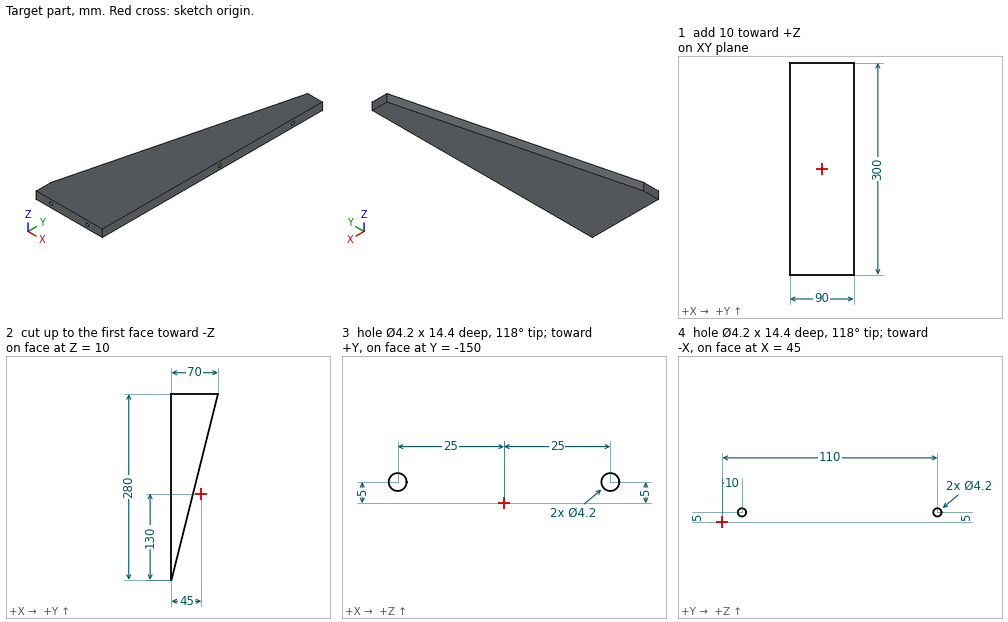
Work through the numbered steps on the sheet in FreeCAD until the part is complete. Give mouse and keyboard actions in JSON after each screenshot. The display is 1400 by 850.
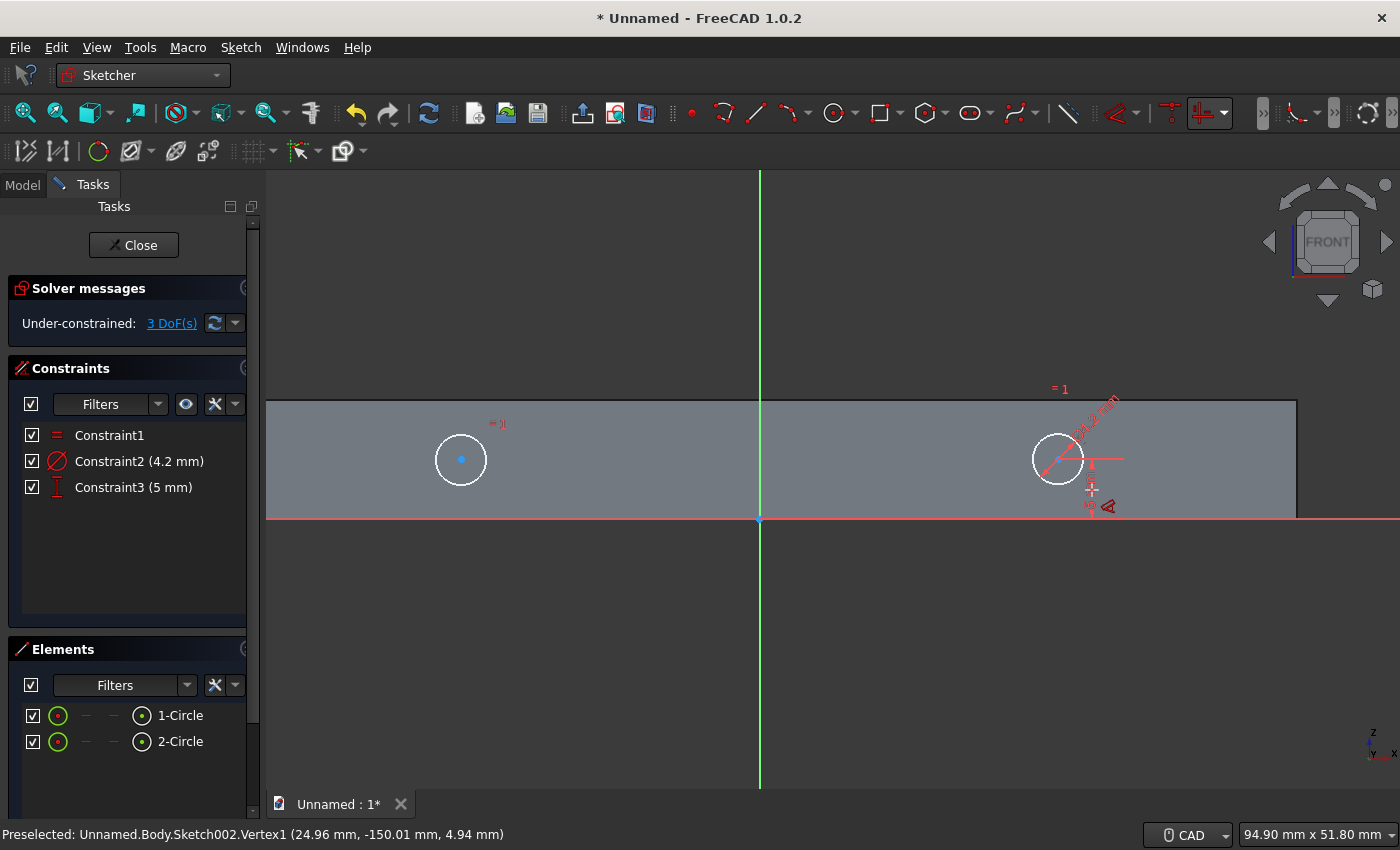
{"action": "left_click", "coordinate": [461, 460]}
{"action": "left_click", "coordinate": [427, 490]}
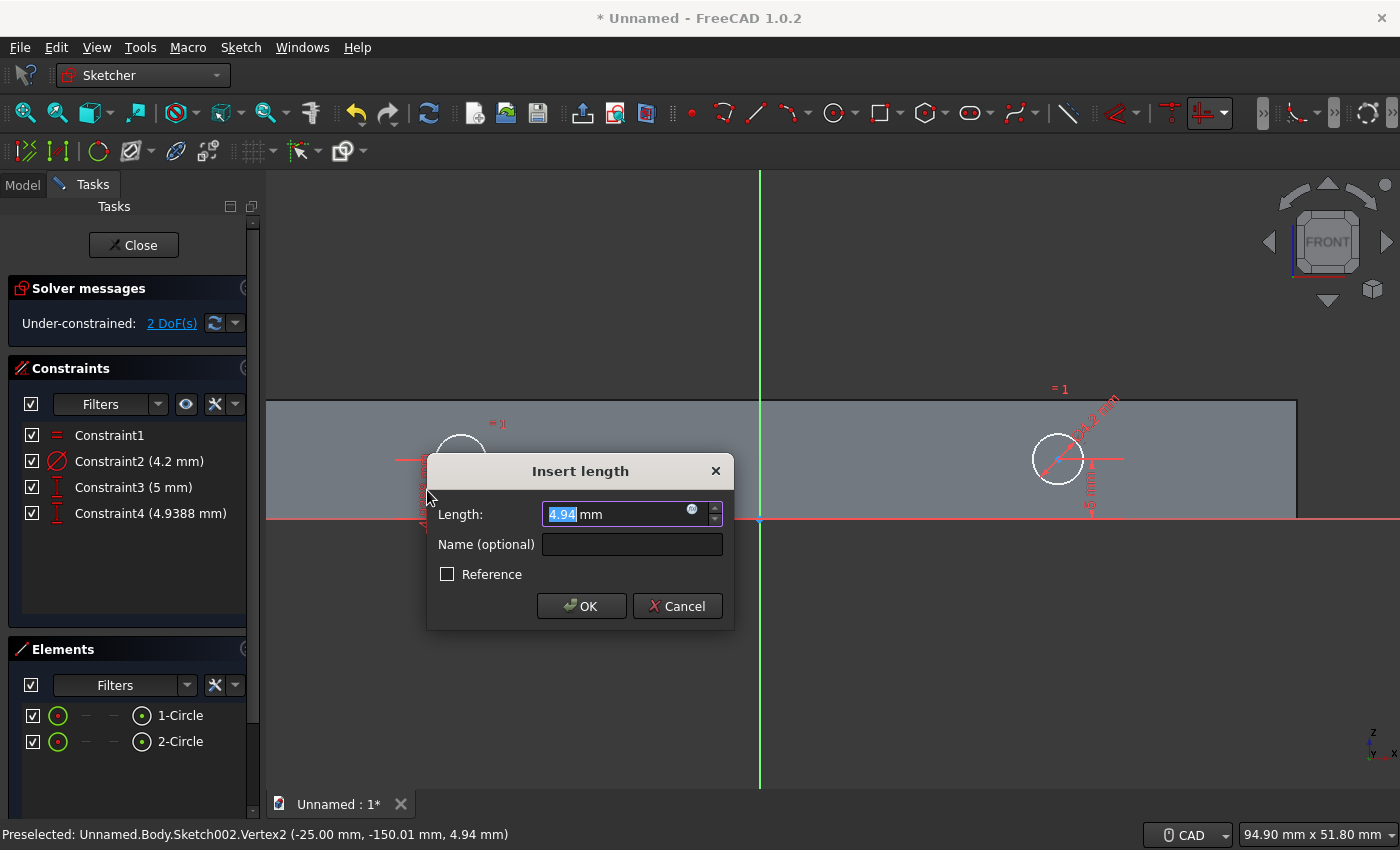
{"action": "type", "text": "5"}
{"action": "key", "text": "Return"}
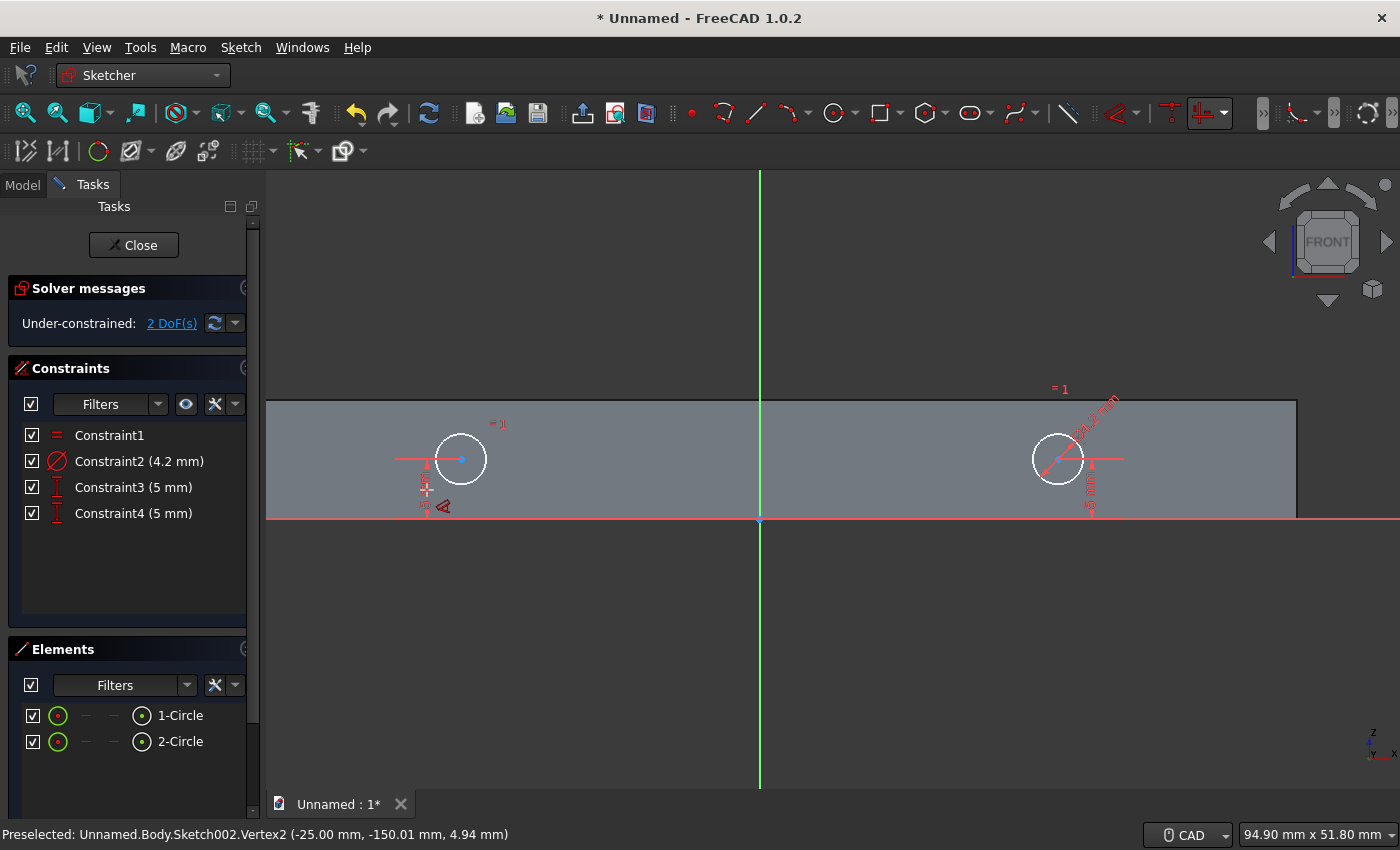
{"action": "left_click", "coordinate": [1058, 459]}
{"action": "left_click", "coordinate": [909, 553]}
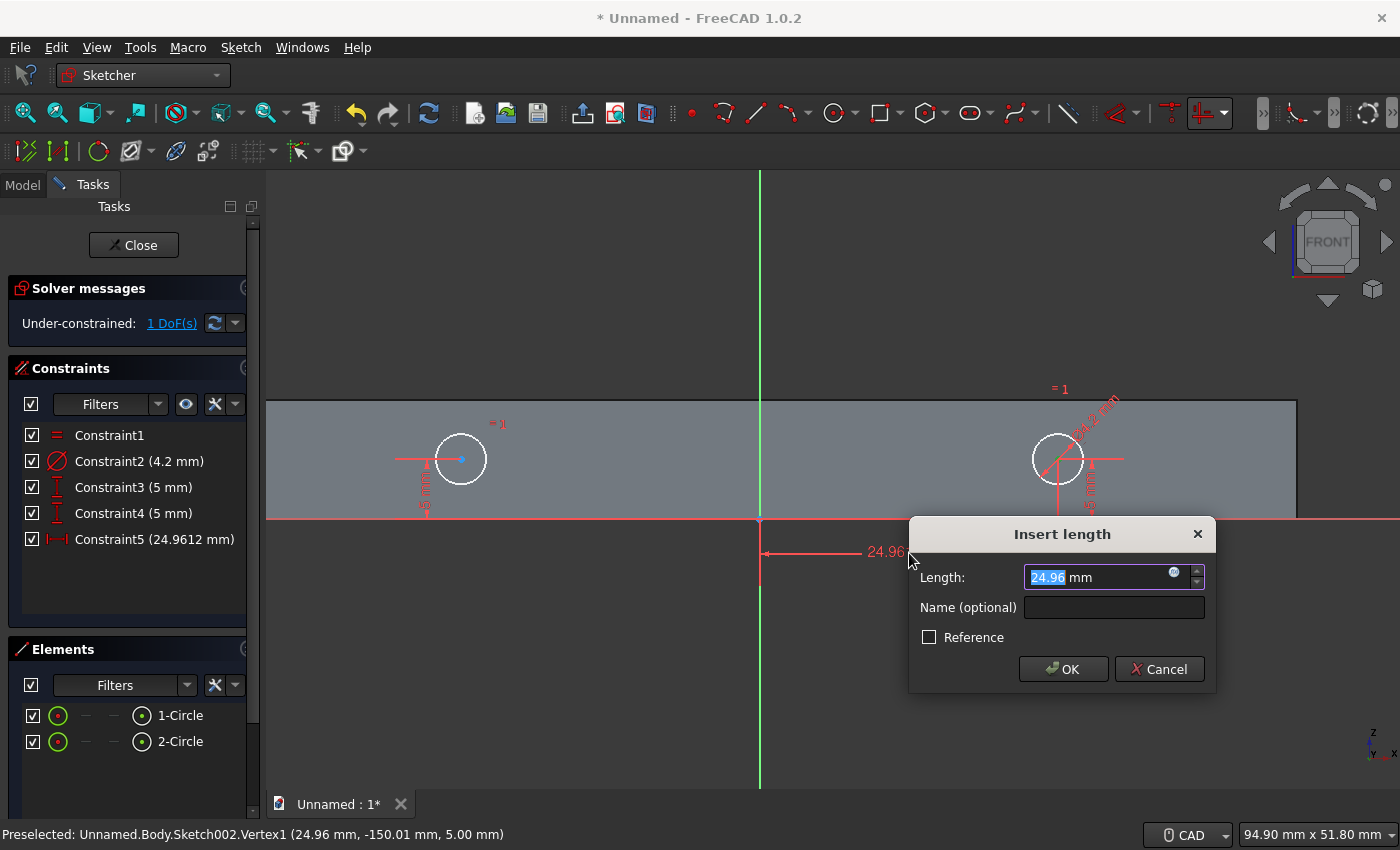
{"action": "type", "text": "25"}
{"action": "key", "text": "Return"}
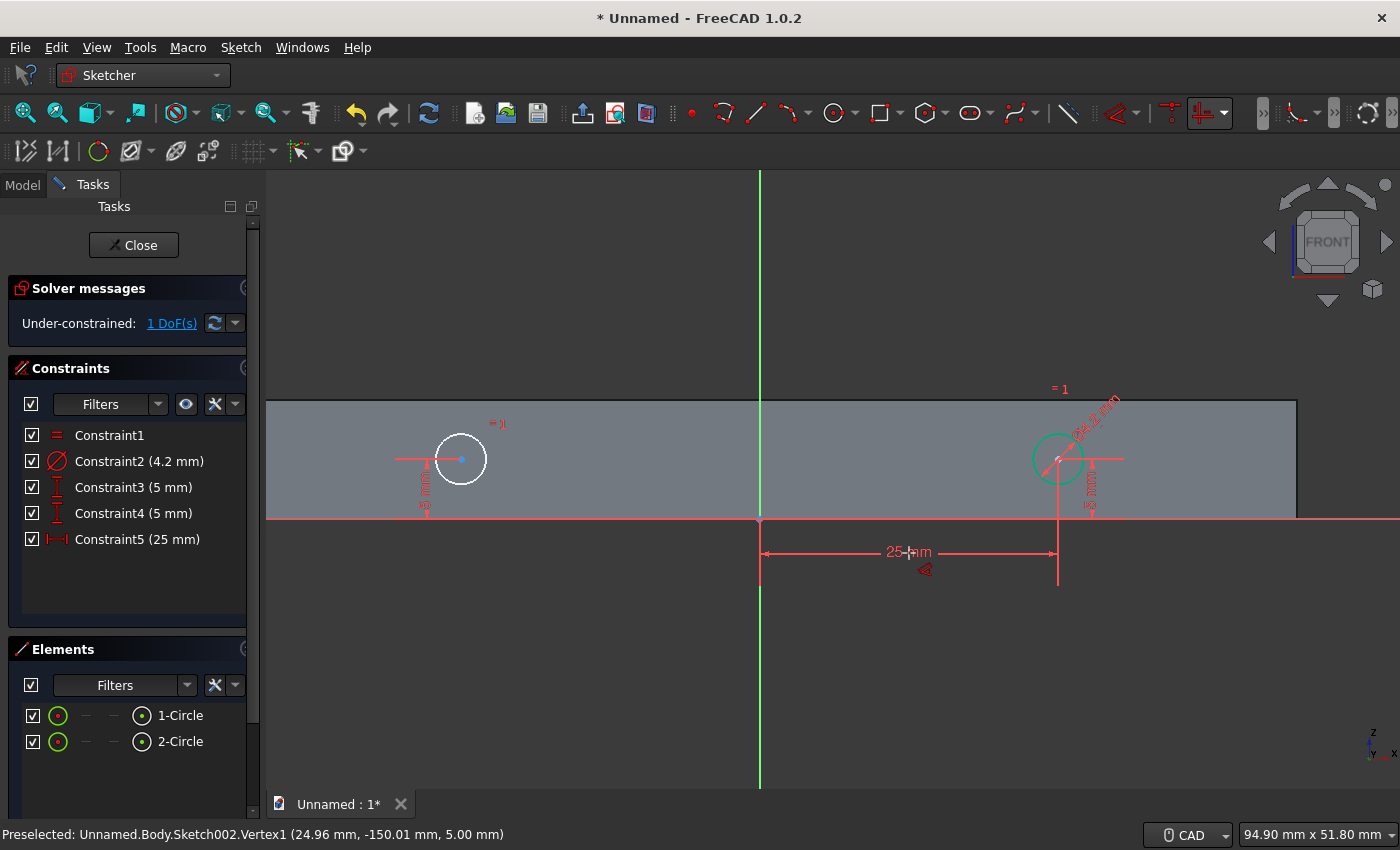
{"action": "left_click", "coordinate": [461, 459]}
{"action": "left_click", "coordinate": [610, 553]}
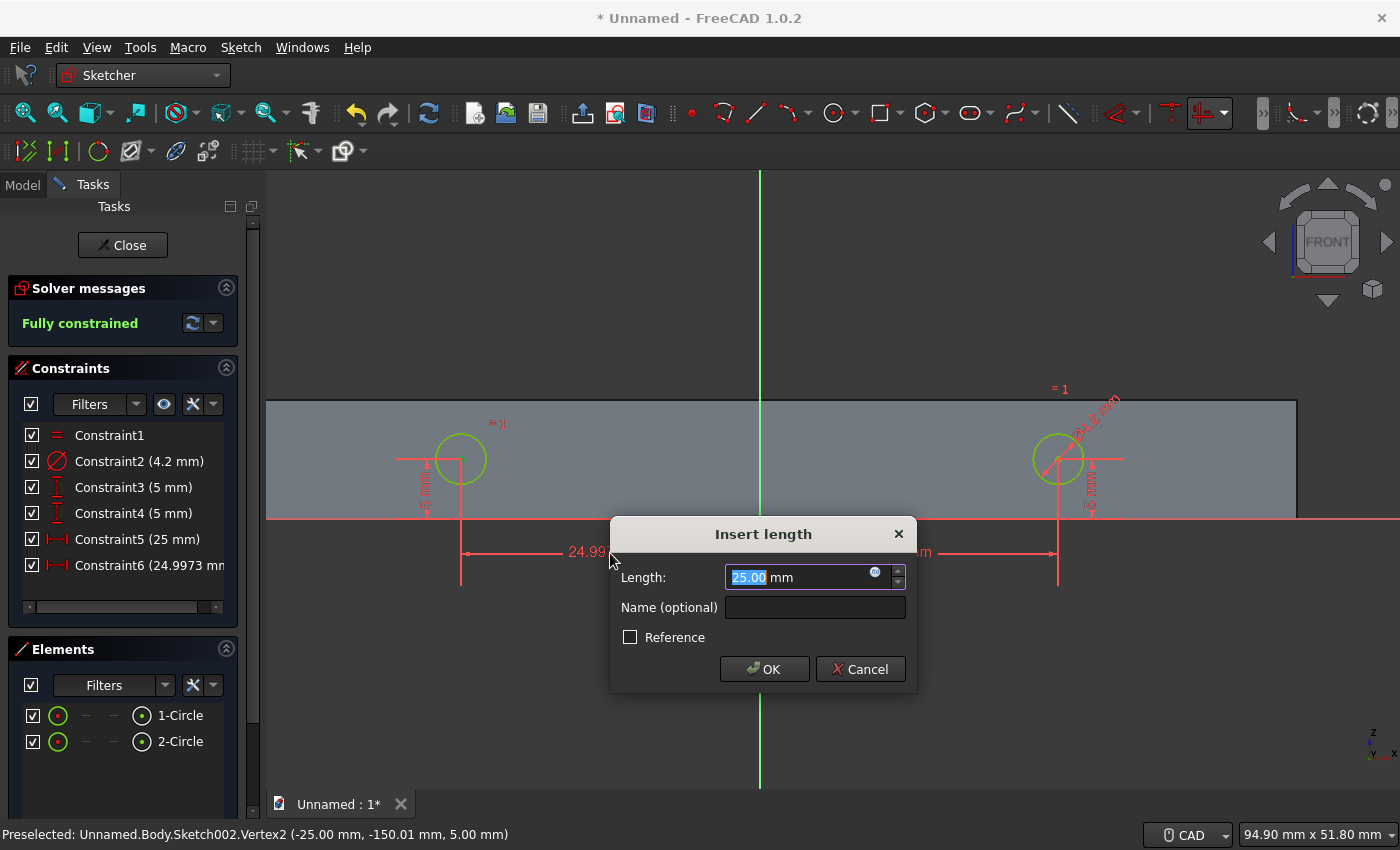
{"action": "type", "text": "25"}
{"action": "key", "text": "Return"}
{"action": "key", "text": "Escape"}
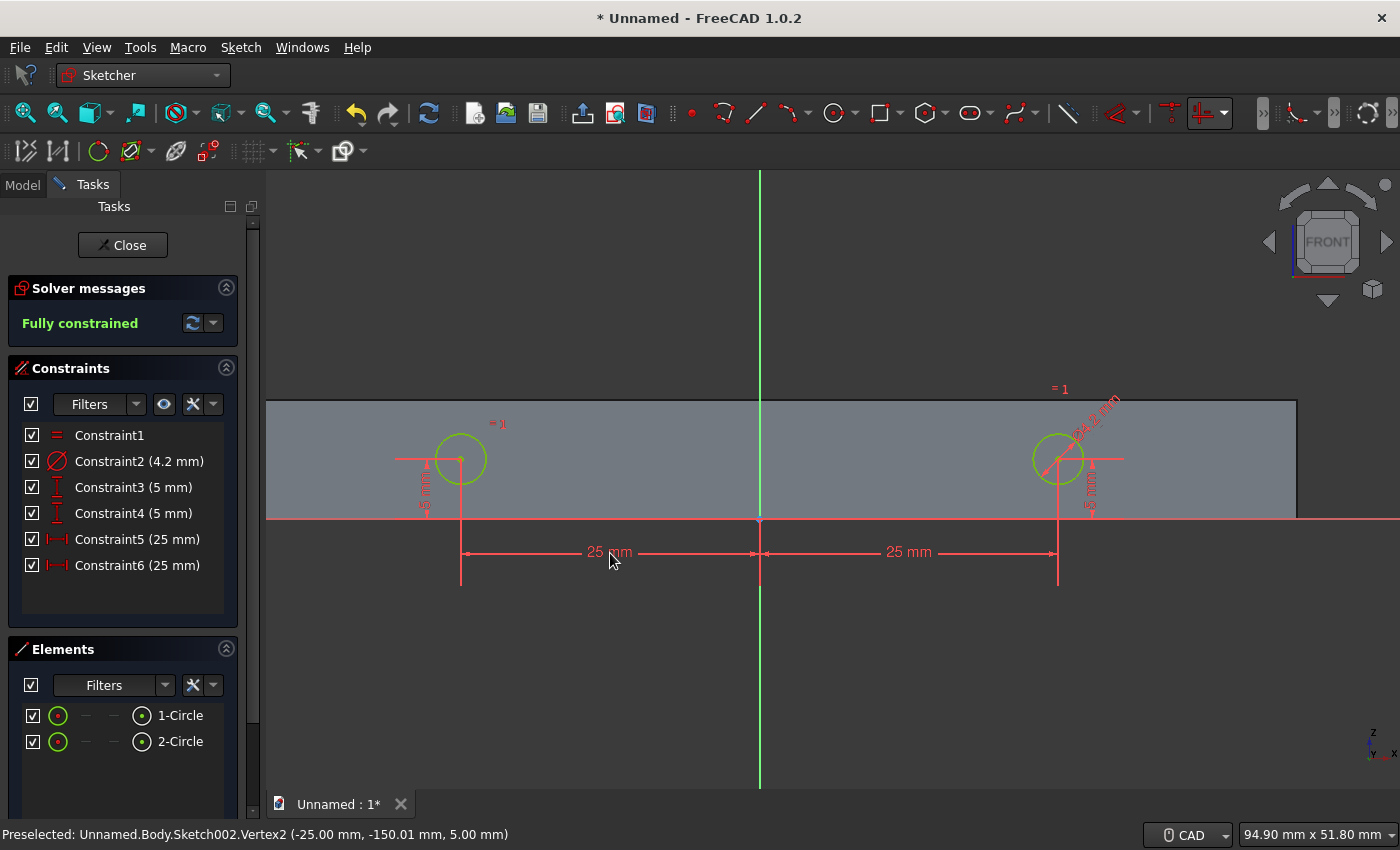
{"action": "left_click", "coordinate": [123, 245]}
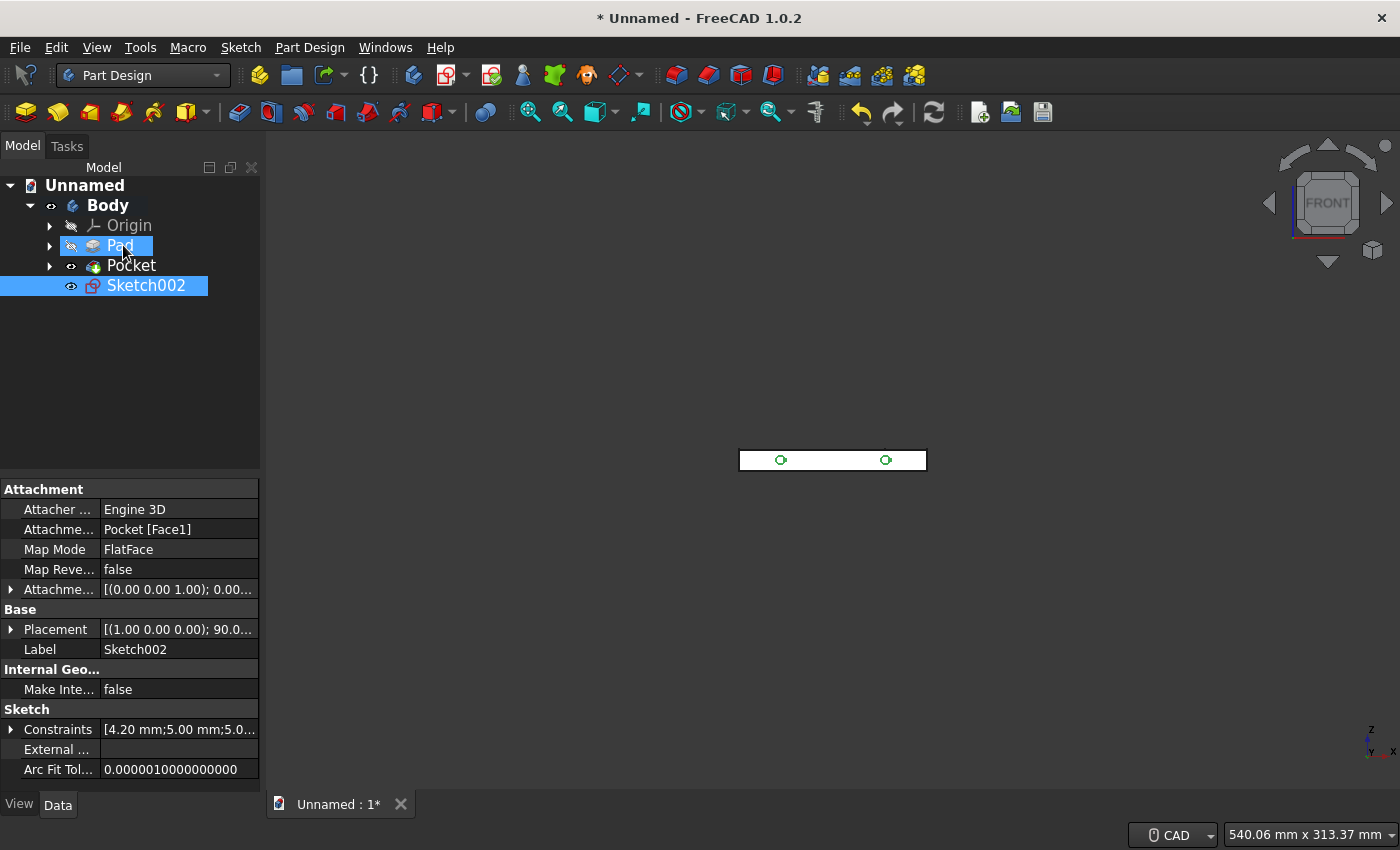
{"action": "left_click", "coordinate": [272, 112]}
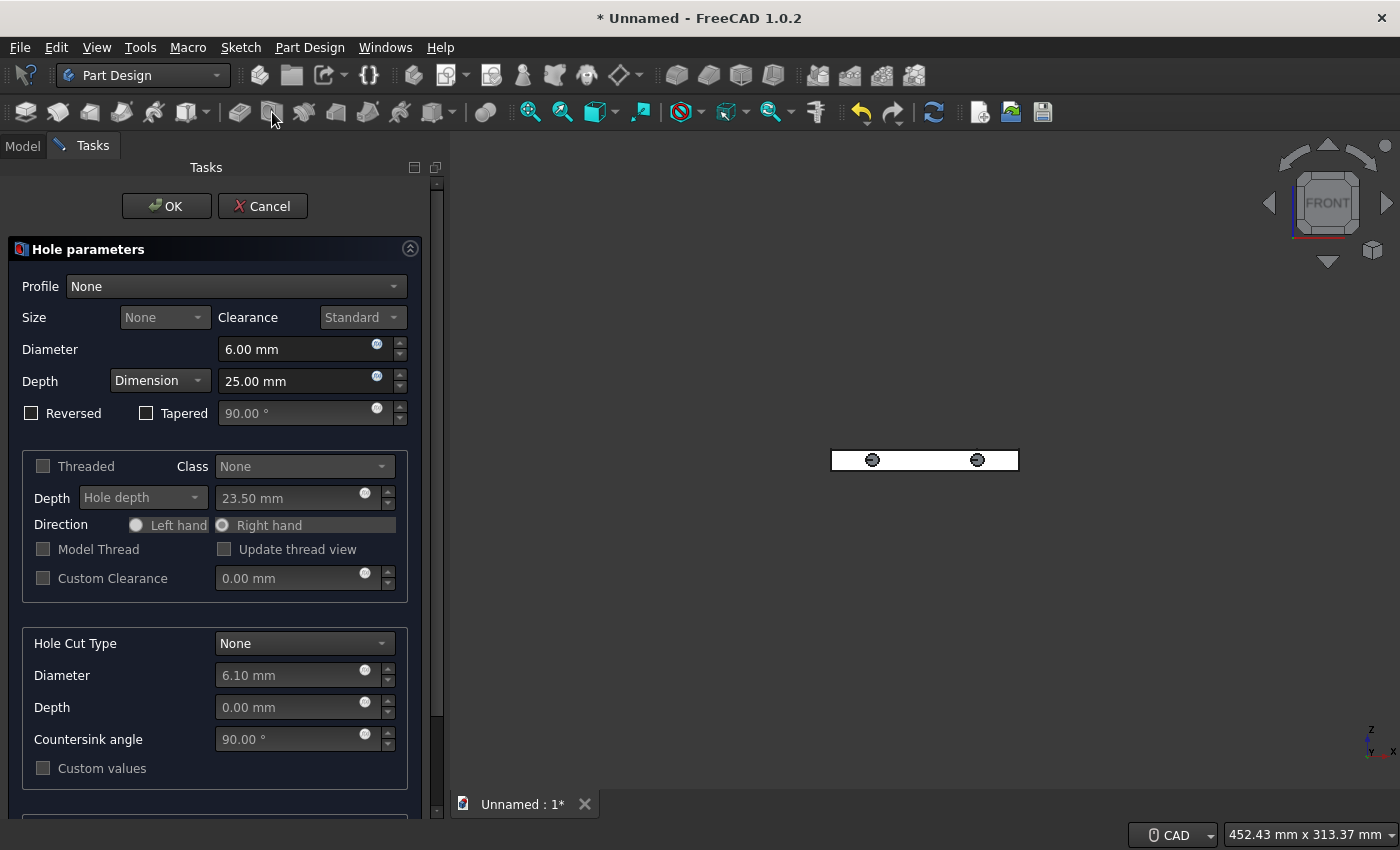
{"action": "triple_click", "coordinate": [305, 349]}